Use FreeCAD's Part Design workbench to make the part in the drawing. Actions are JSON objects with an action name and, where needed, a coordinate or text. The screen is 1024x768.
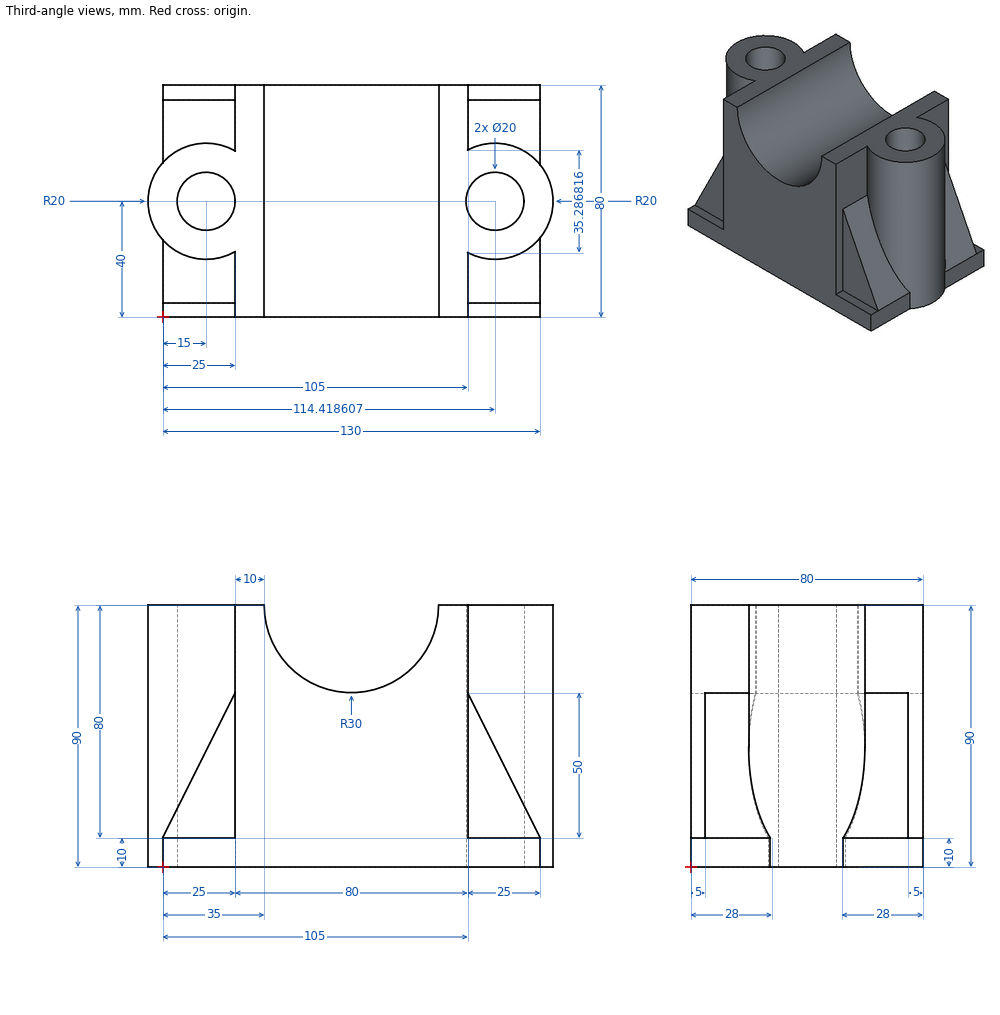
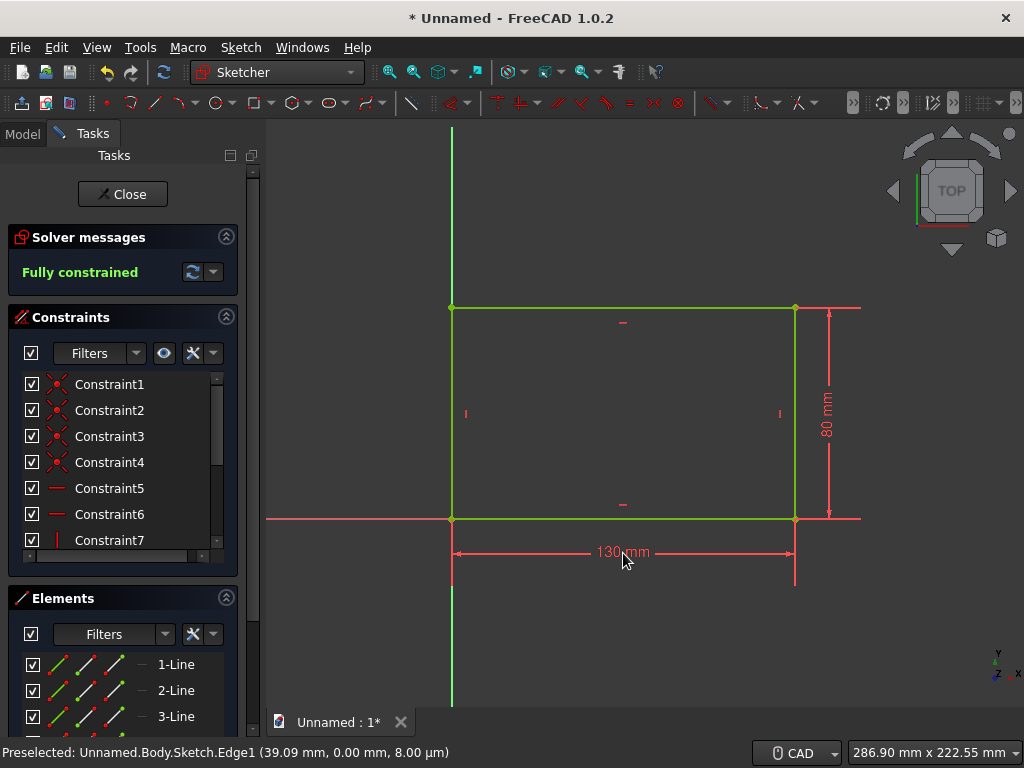
{"action": "left_click", "coordinate": [123, 194]}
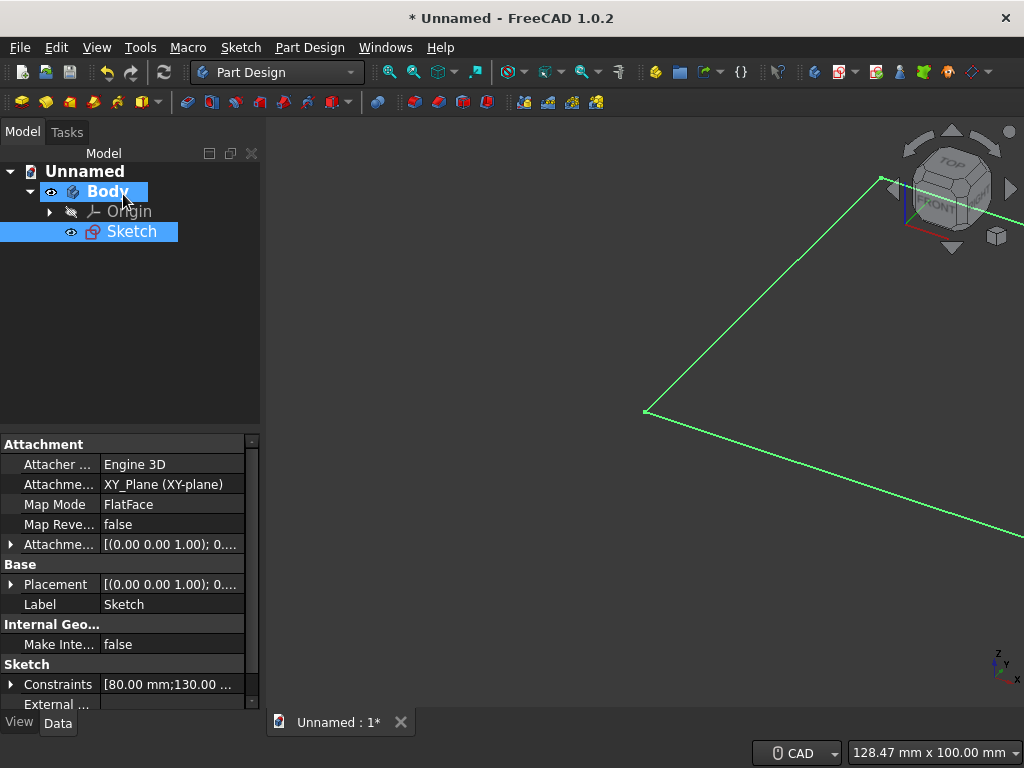
{"action": "left_click", "coordinate": [22, 102]}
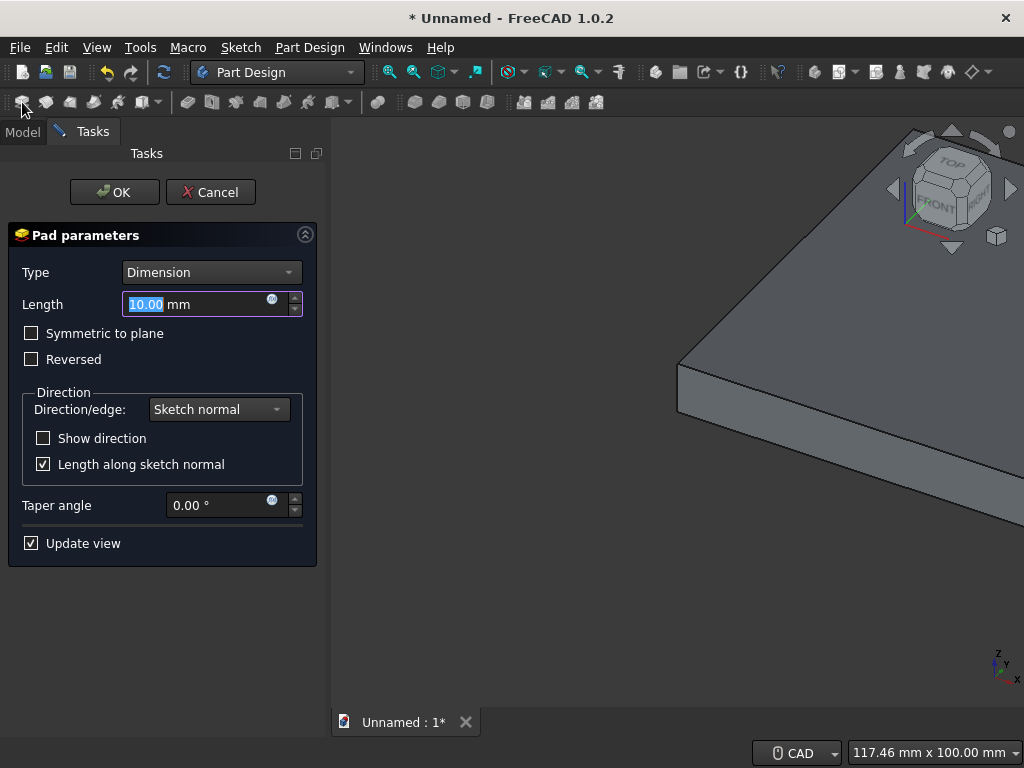
{"action": "type", "text": "10"}
{"action": "key", "text": "Tab"}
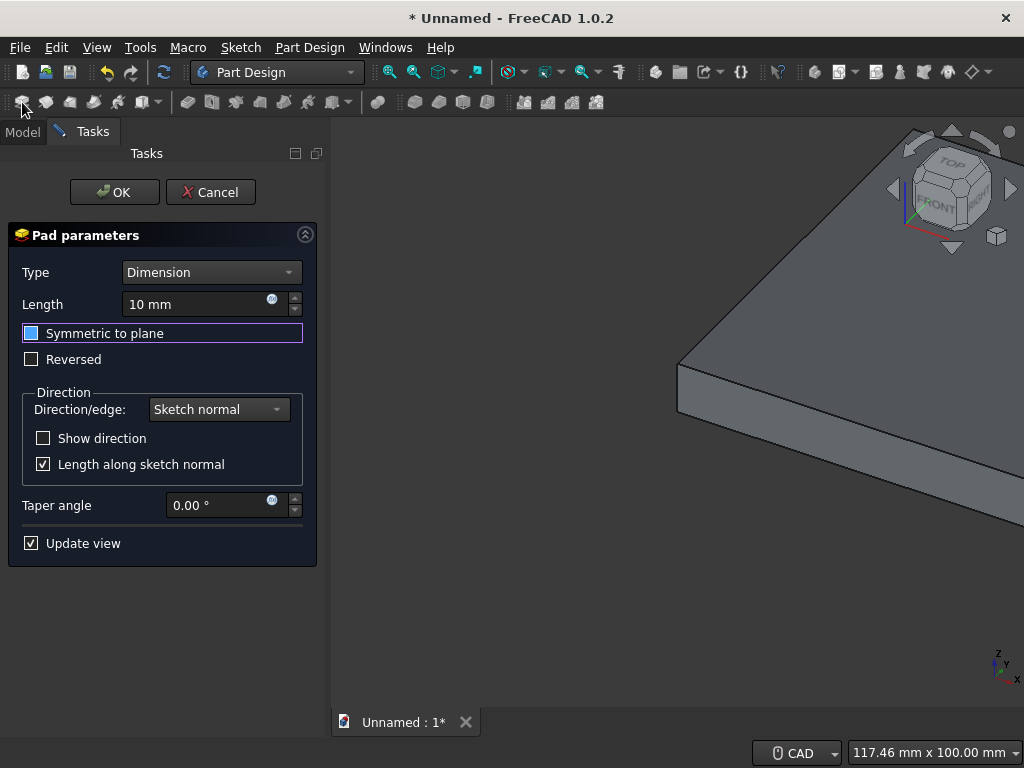
{"action": "left_click", "coordinate": [115, 192]}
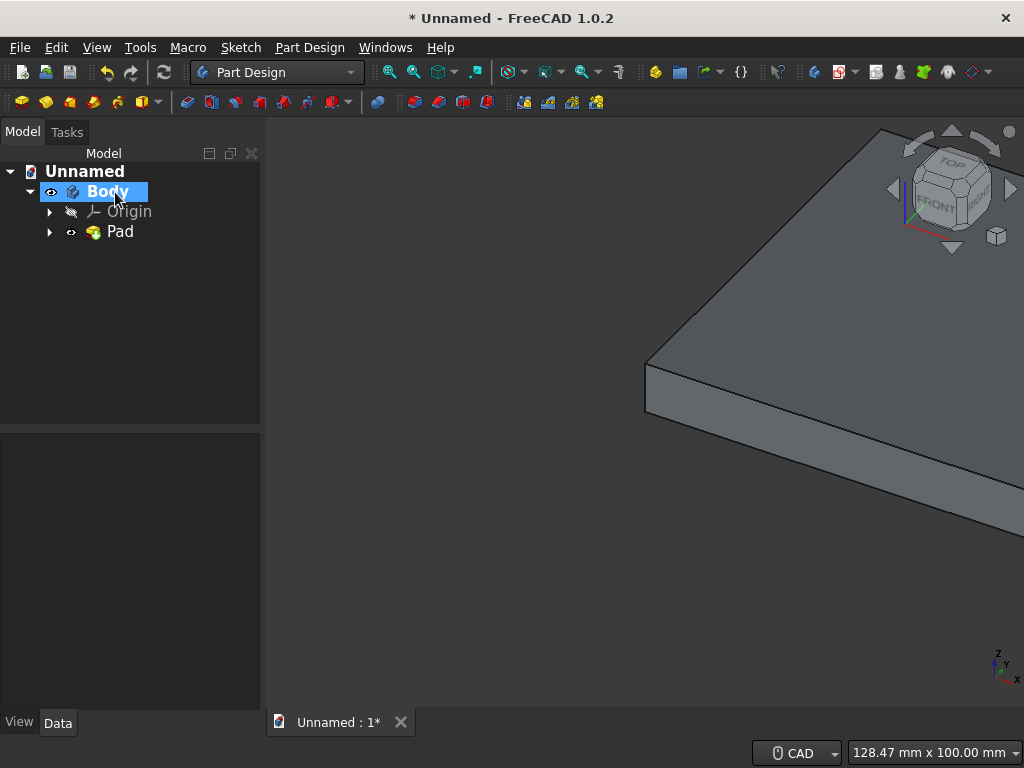
{"action": "left_click", "coordinate": [390, 72]}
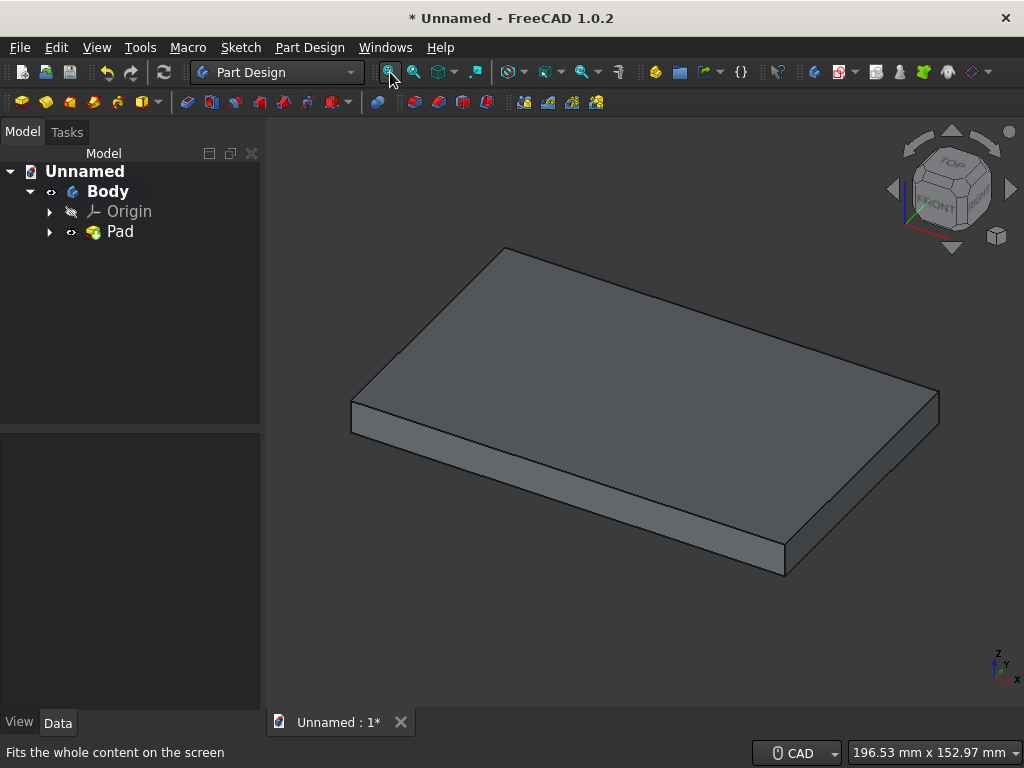
{"action": "left_click", "coordinate": [754, 549]}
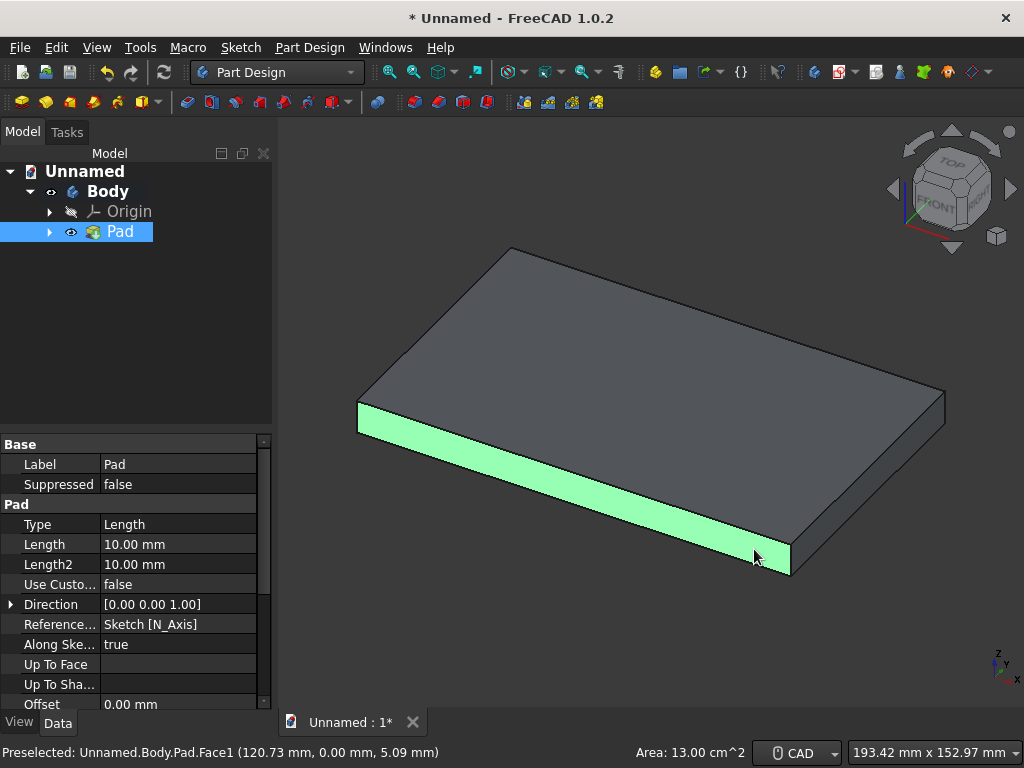
{"action": "left_click", "coordinate": [840, 72]}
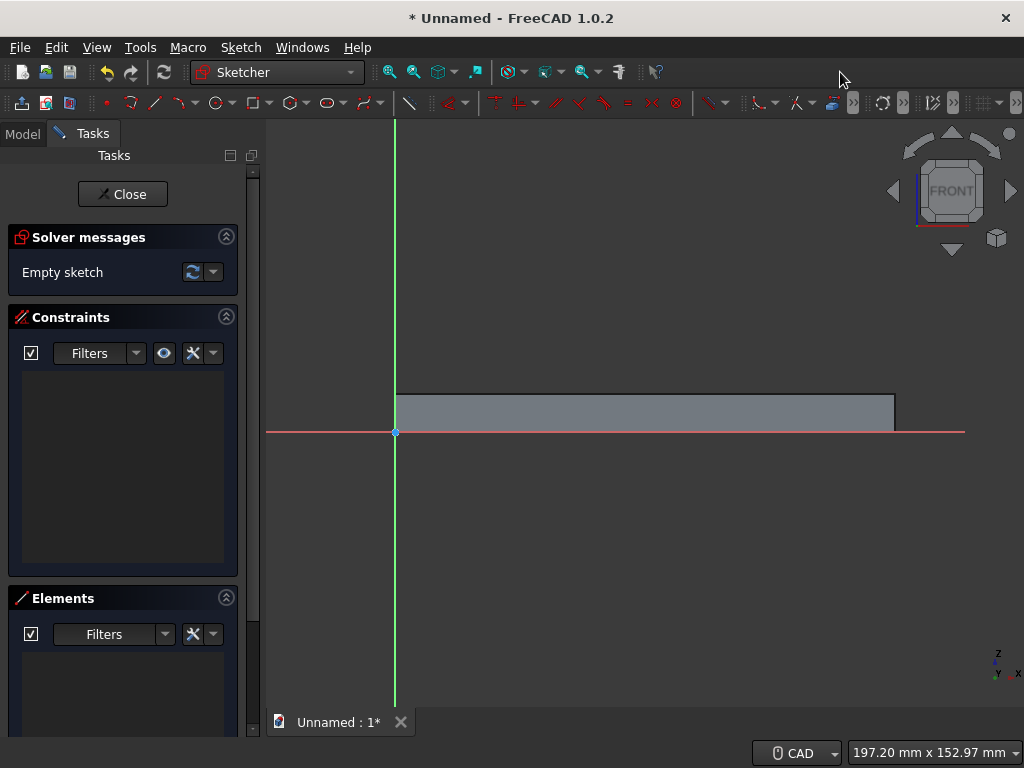
{"action": "scroll", "coordinate": [484, 679], "scroll_direction": "down", "scroll_amount": 1}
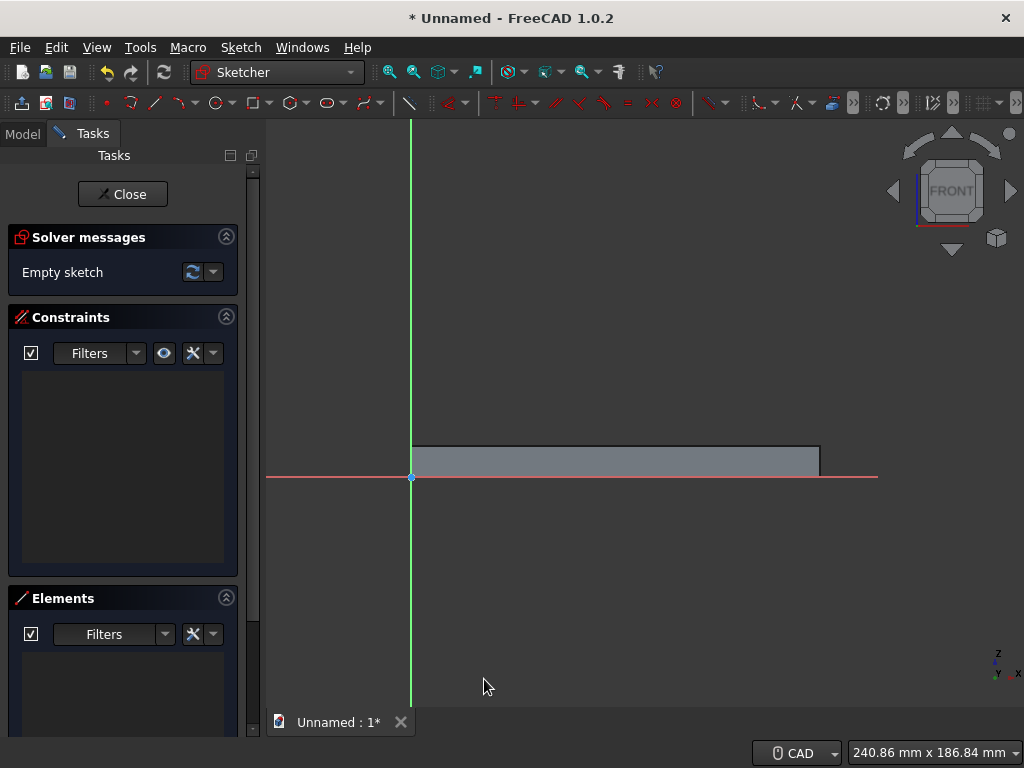
{"action": "left_click", "coordinate": [132, 104]}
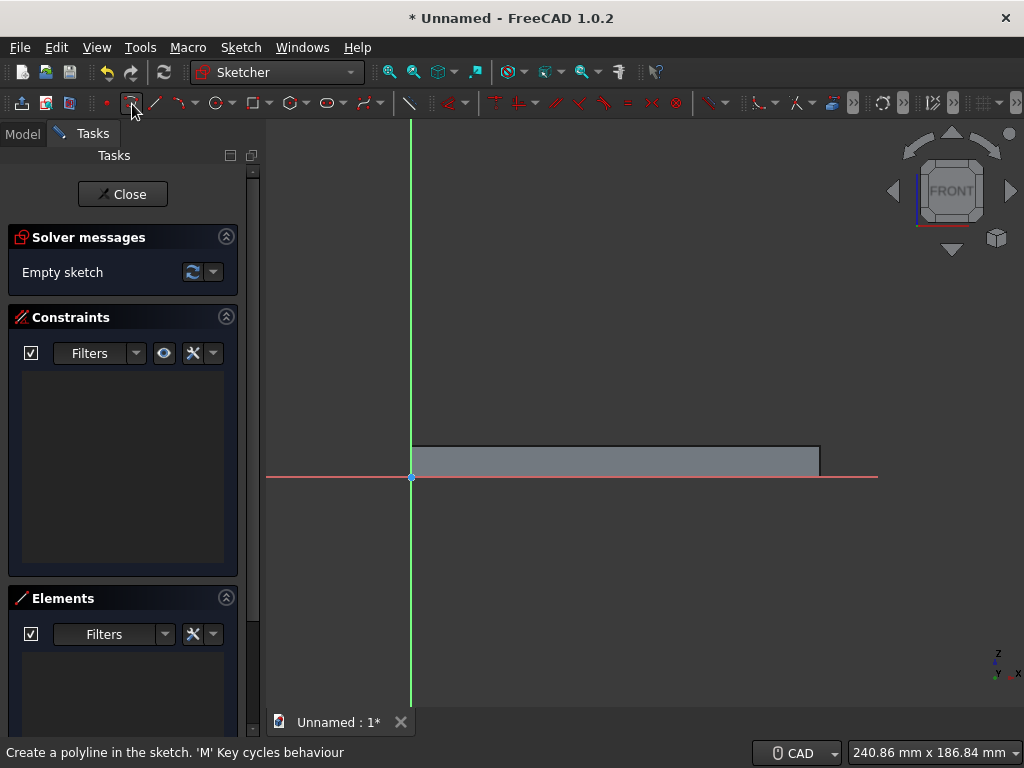
{"action": "left_click", "coordinate": [521, 194]}
{"action": "left_click", "coordinate": [490, 194]}
{"action": "left_click", "coordinate": [490, 446]}
{"action": "left_click", "coordinate": [742, 446]}
{"action": "left_click", "coordinate": [742, 194]}
{"action": "left_click", "coordinate": [710, 194]}
{"action": "right_click", "coordinate": [710, 194]}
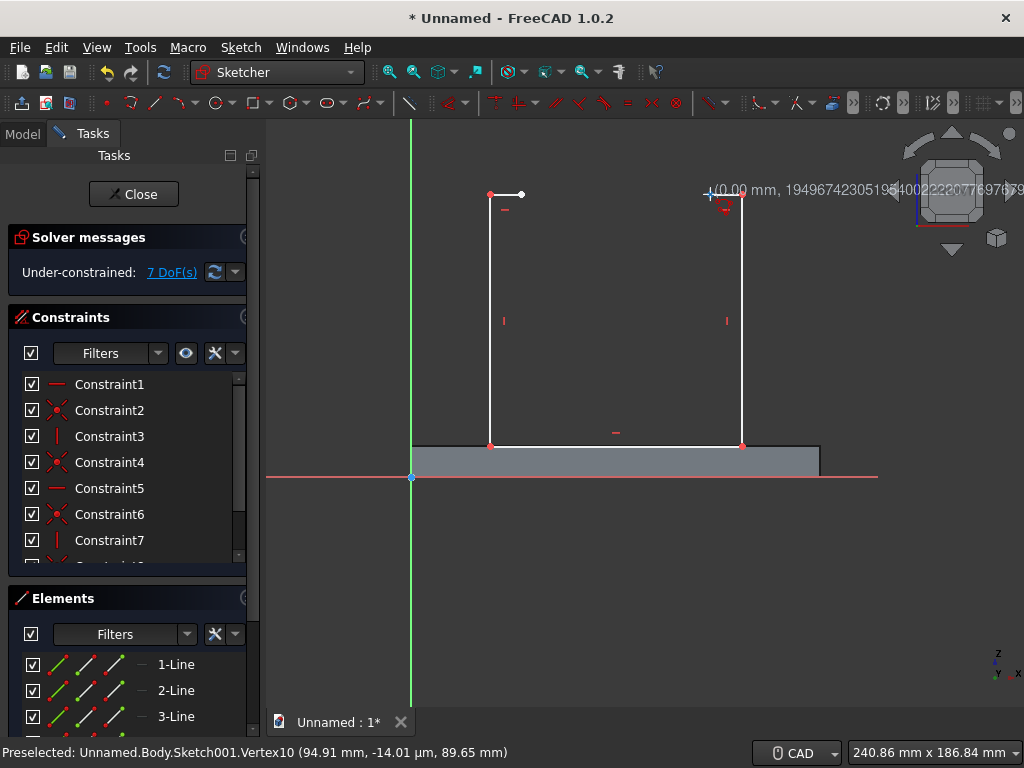
{"action": "left_click", "coordinate": [180, 104]}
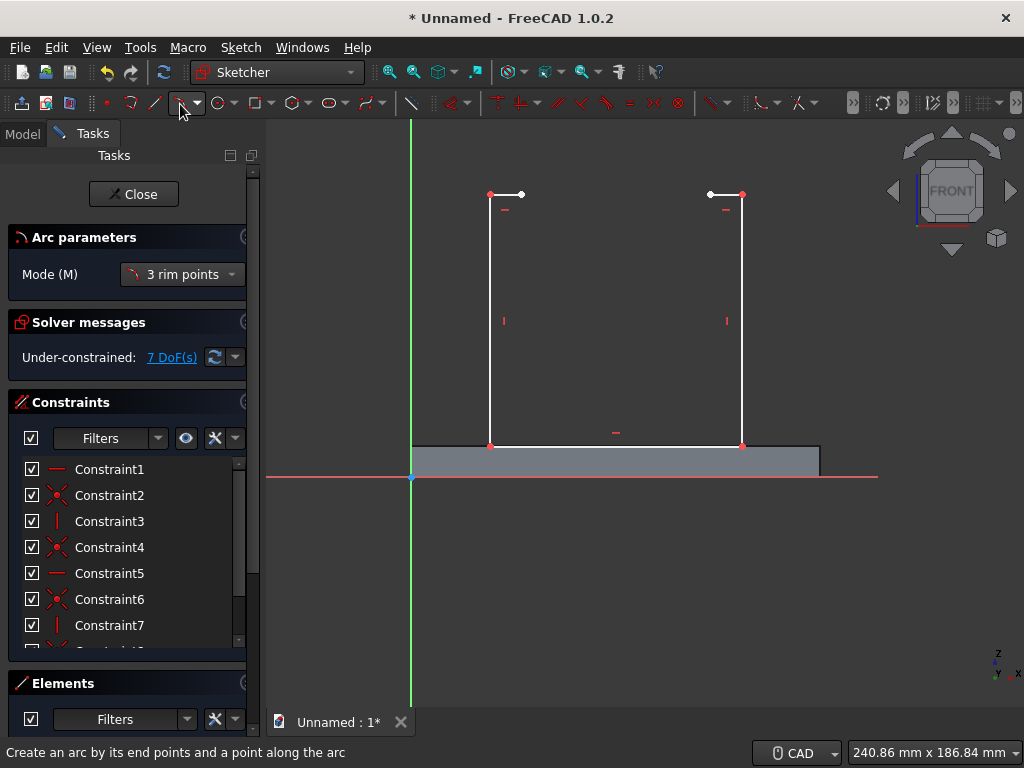
{"action": "left_click", "coordinate": [710, 195]}
{"action": "left_click", "coordinate": [521, 195]}
{"action": "left_click", "coordinate": [616, 288]}
{"action": "key", "text": "Escape"}